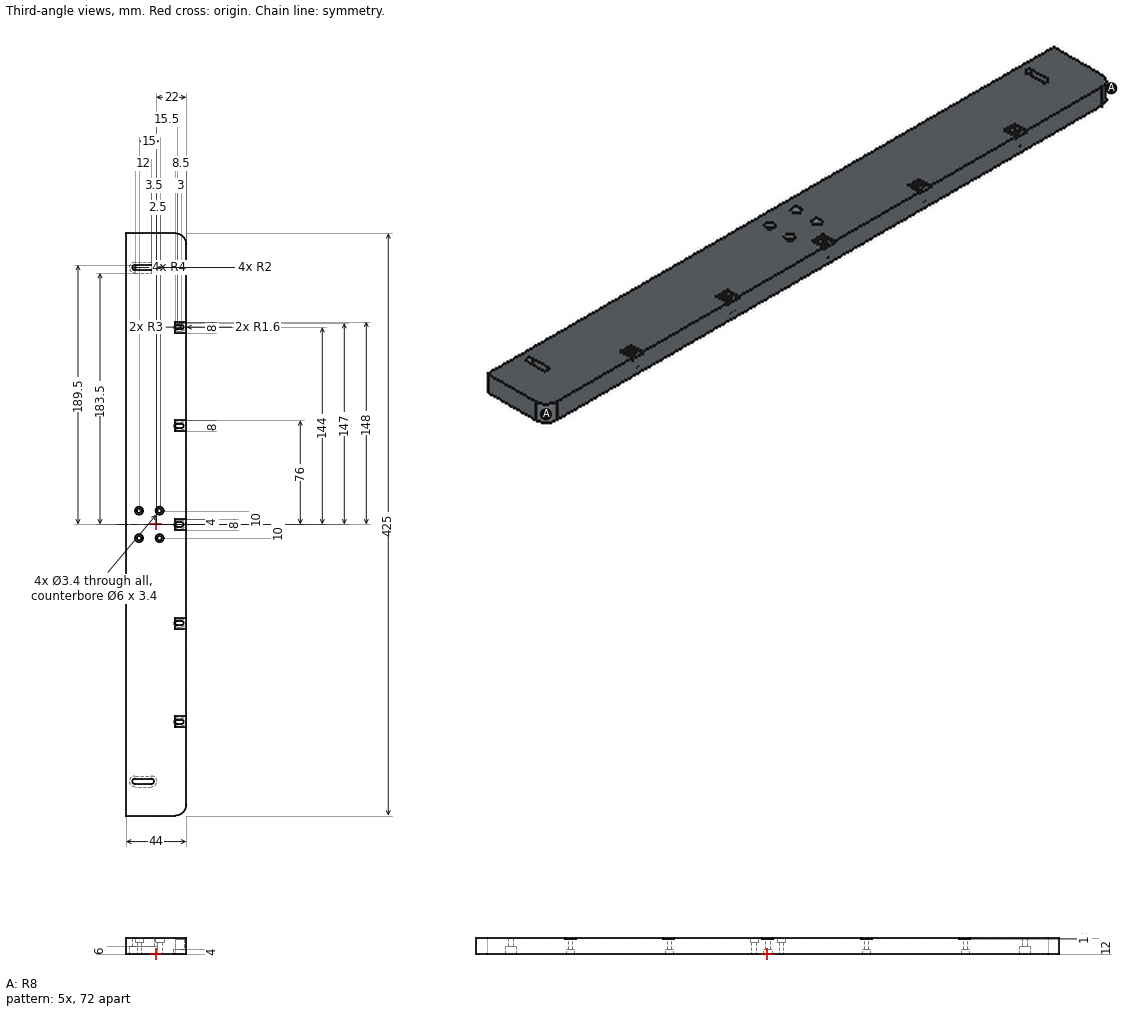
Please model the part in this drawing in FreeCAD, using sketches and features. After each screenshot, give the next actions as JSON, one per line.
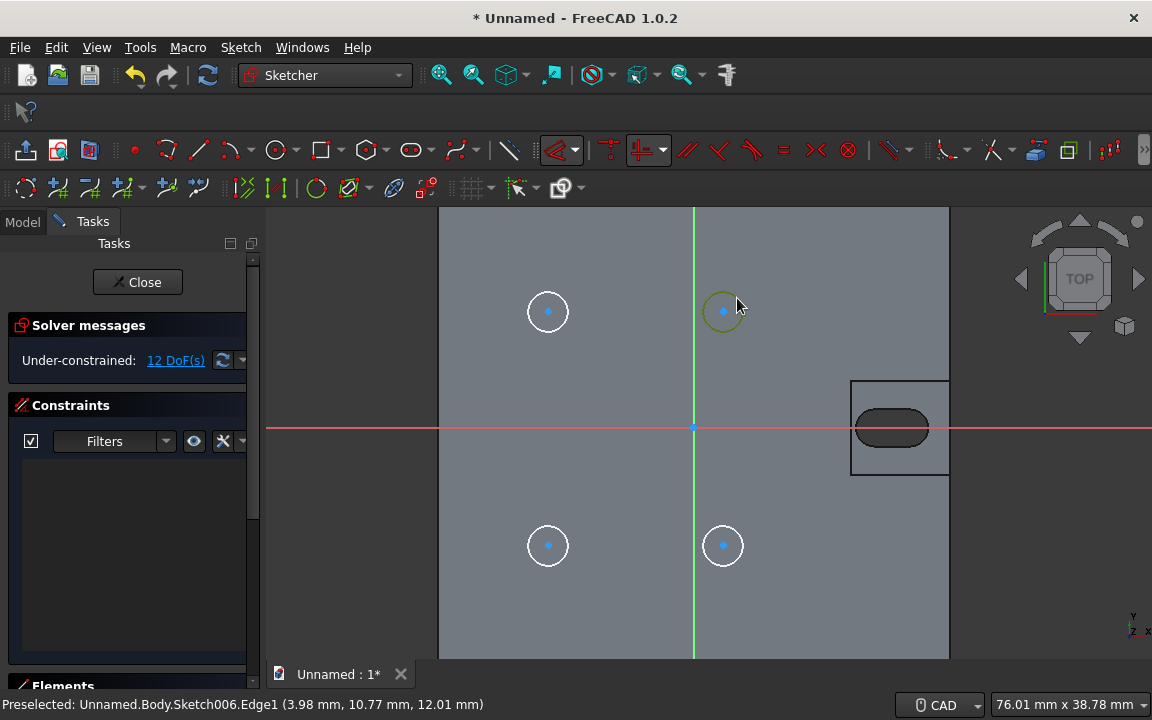
{"action": "left_click", "coordinate": [562, 298]}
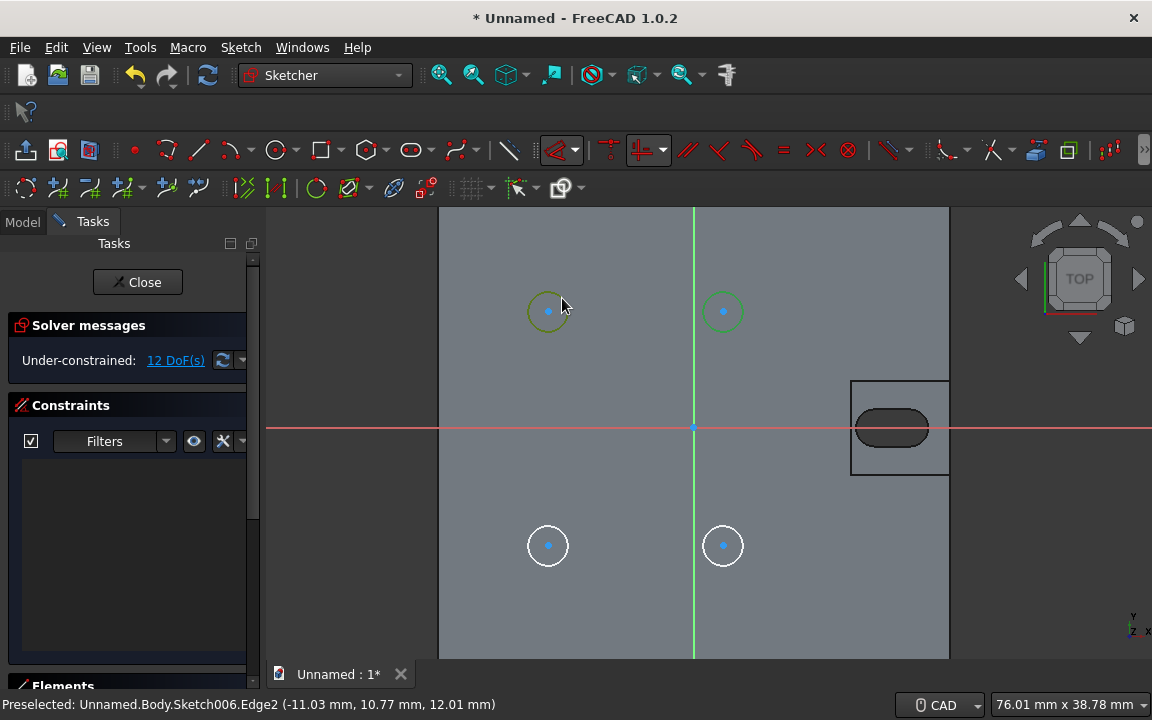
{"action": "left_click", "coordinate": [737, 532]}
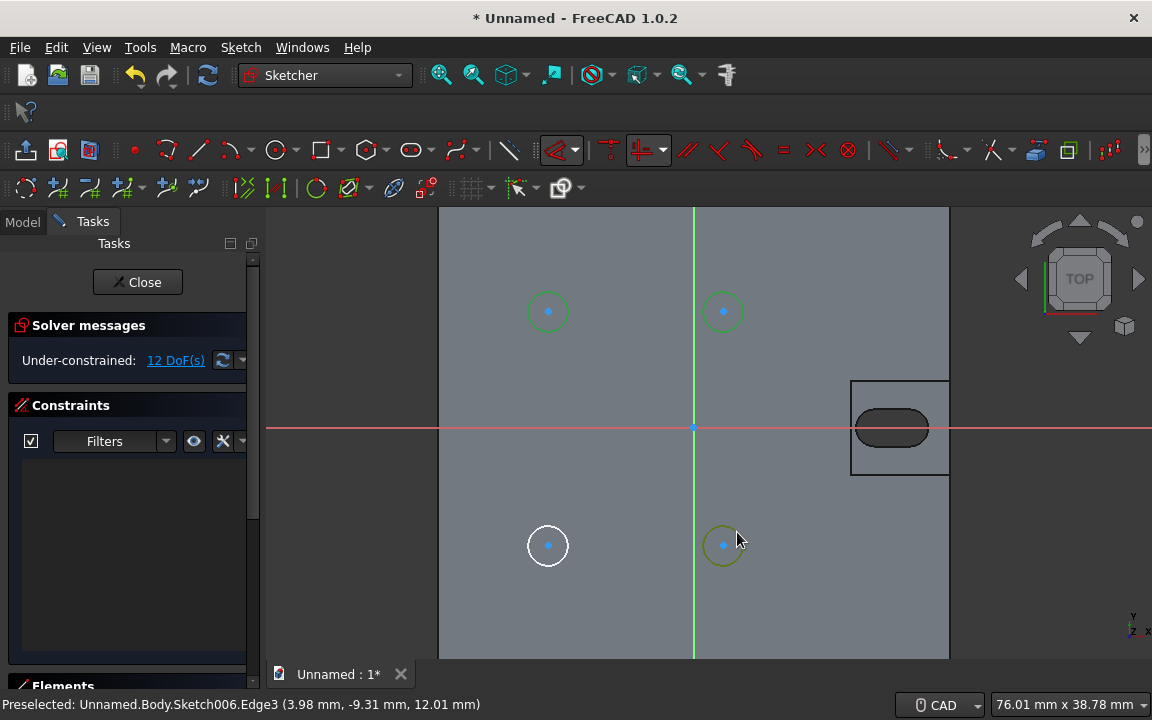
{"action": "left_click", "coordinate": [562, 532]}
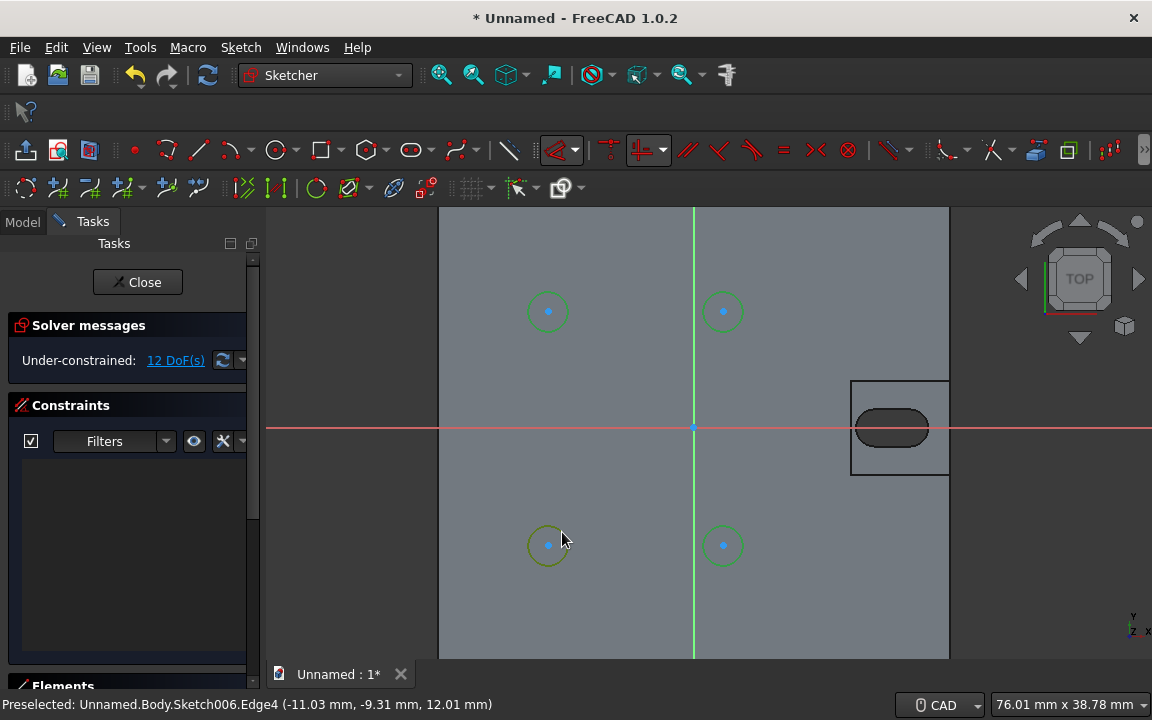
{"action": "left_click", "coordinate": [784, 150]}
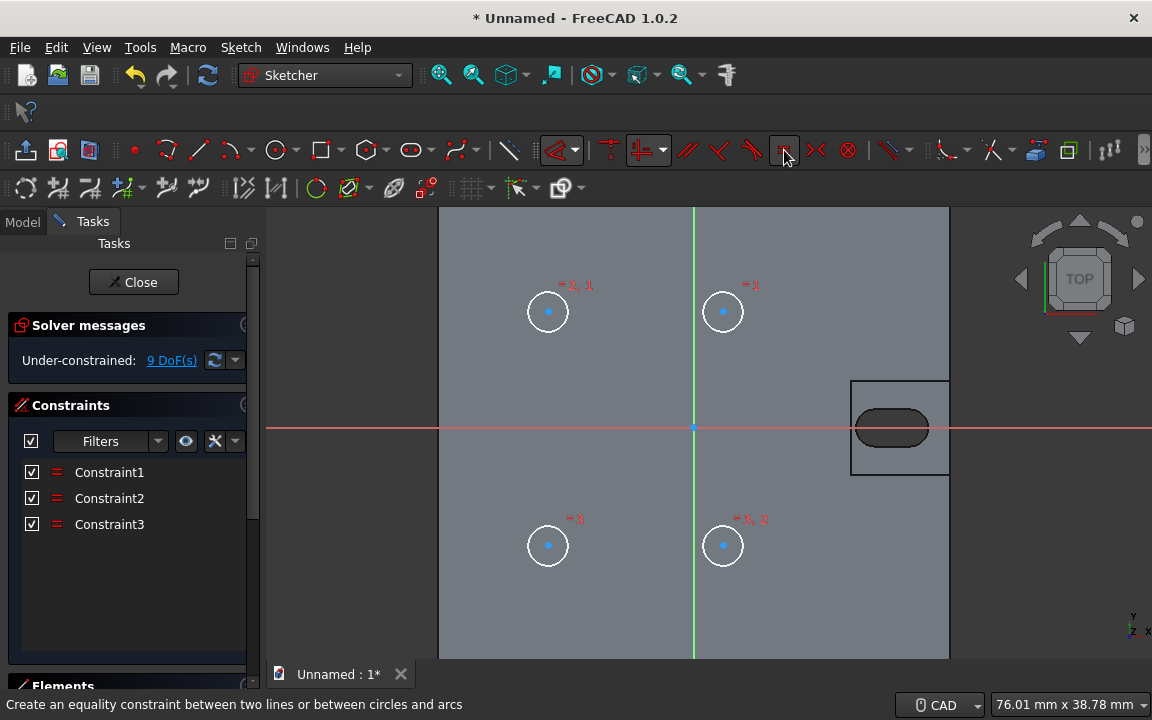
{"action": "left_click", "coordinate": [723, 312]}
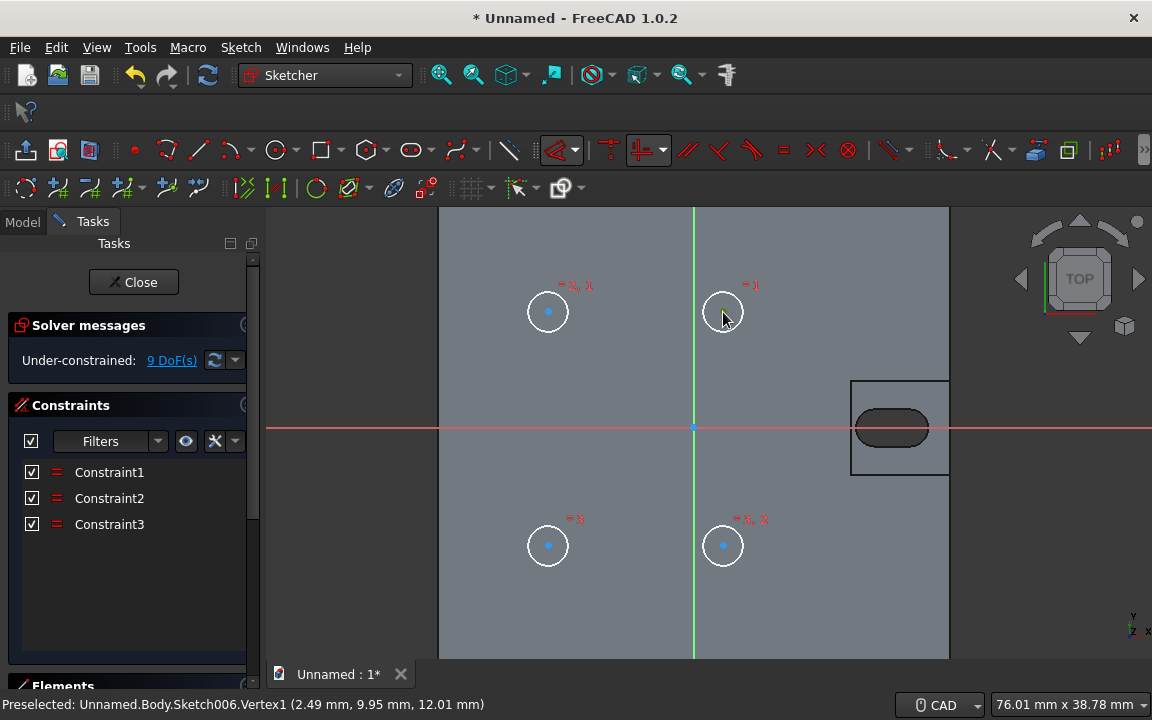
{"action": "left_click", "coordinate": [548, 312]}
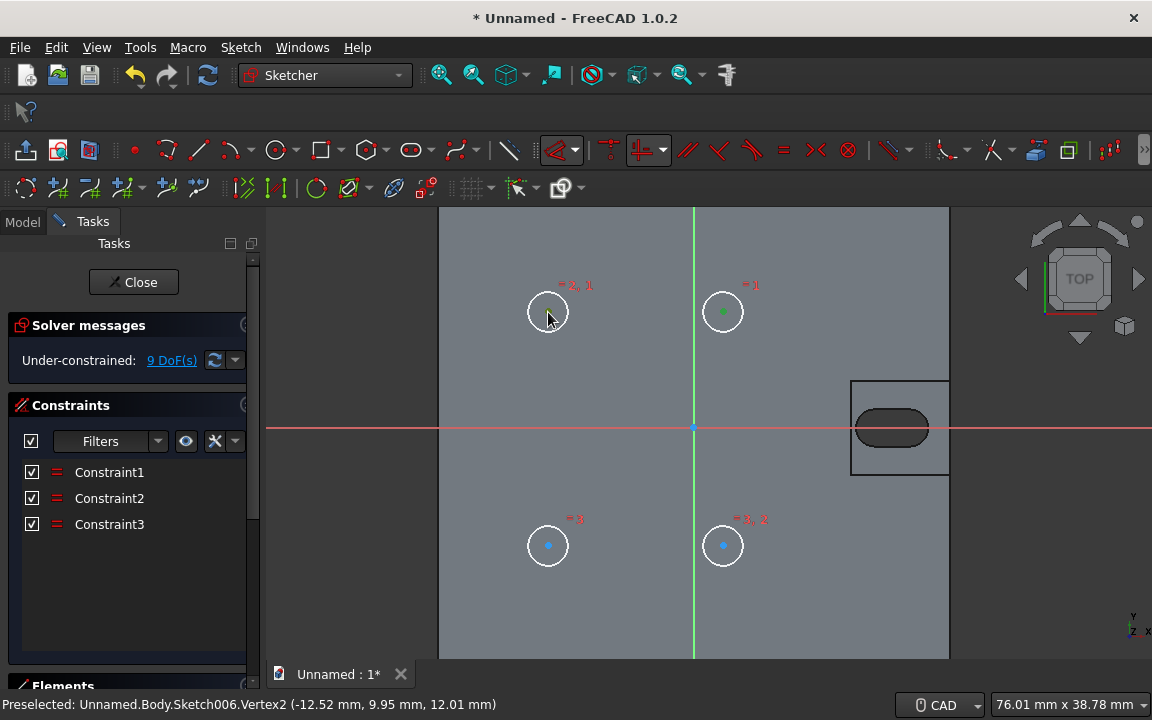
{"action": "key", "text": "h"}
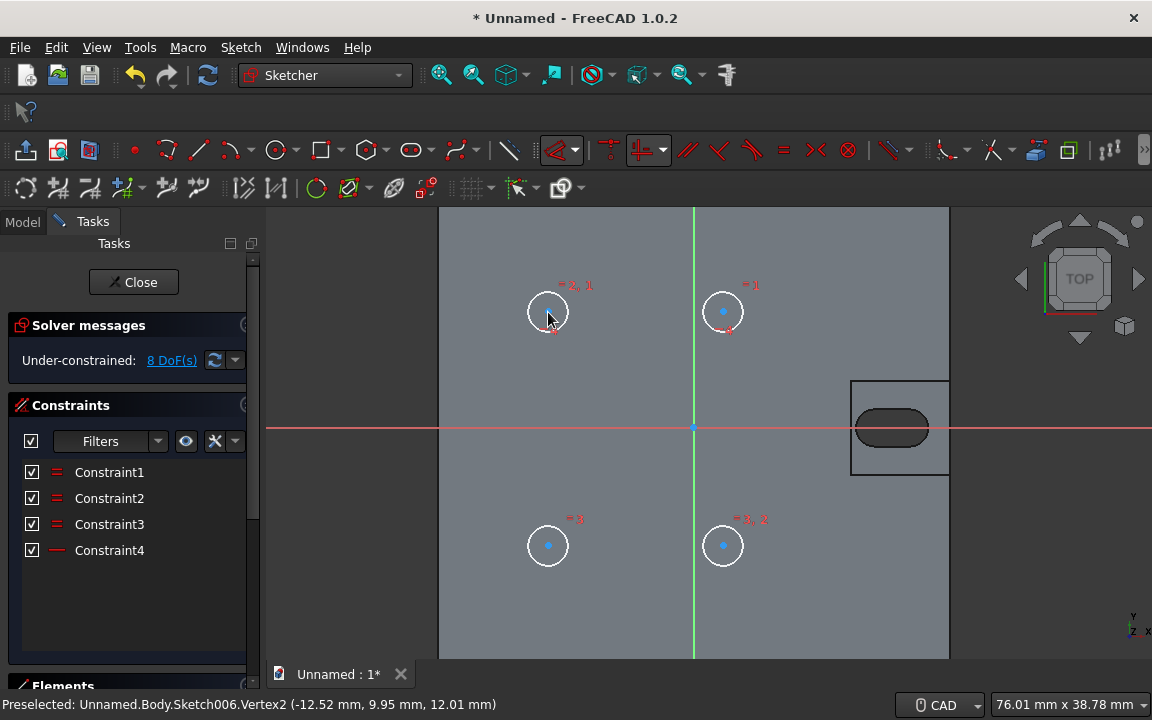
{"action": "left_click", "coordinate": [723, 312]}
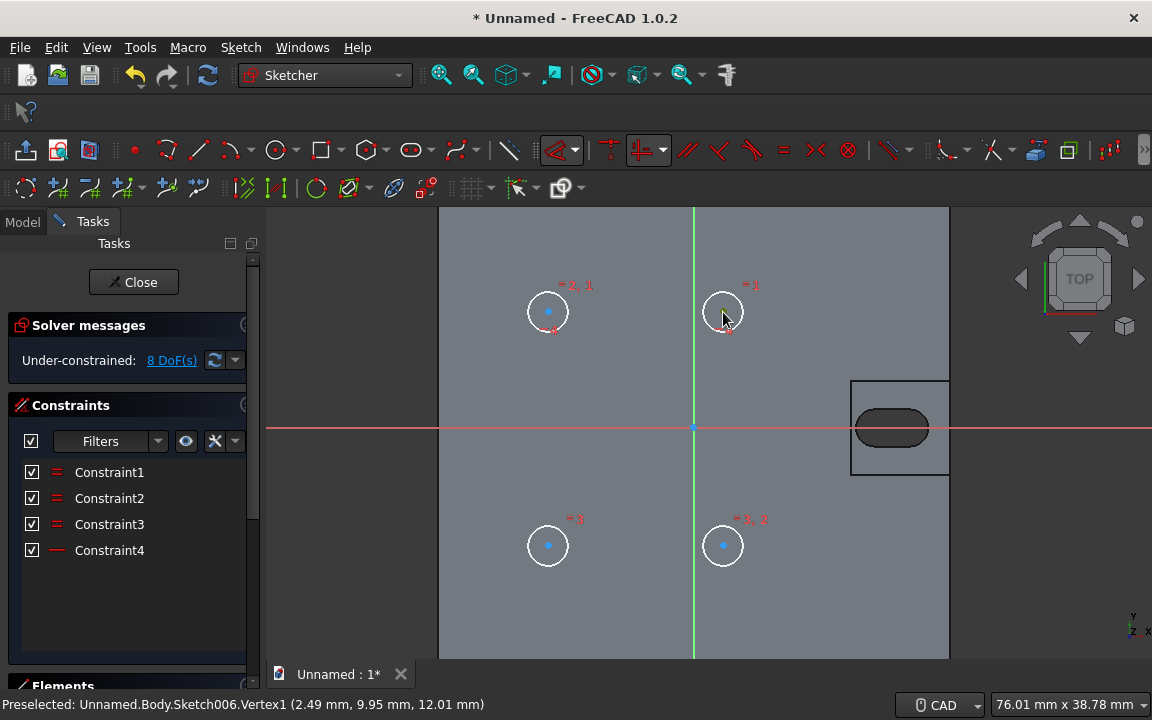
{"action": "left_click", "coordinate": [723, 546]}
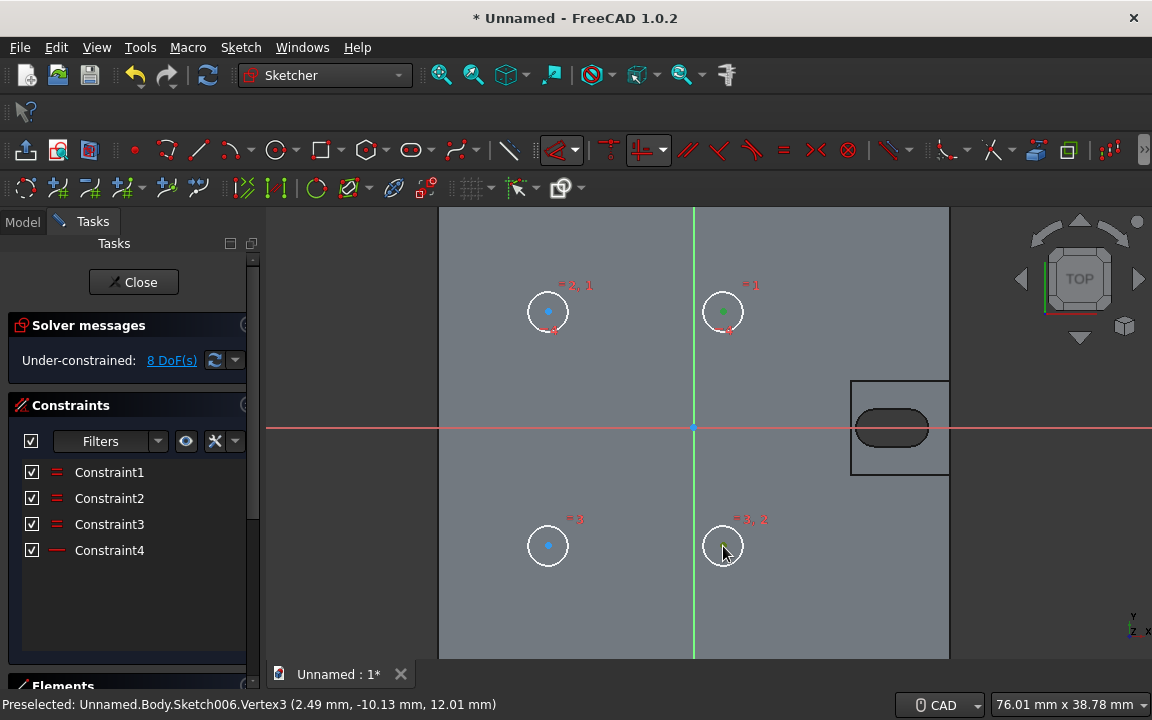
{"action": "key", "text": "v"}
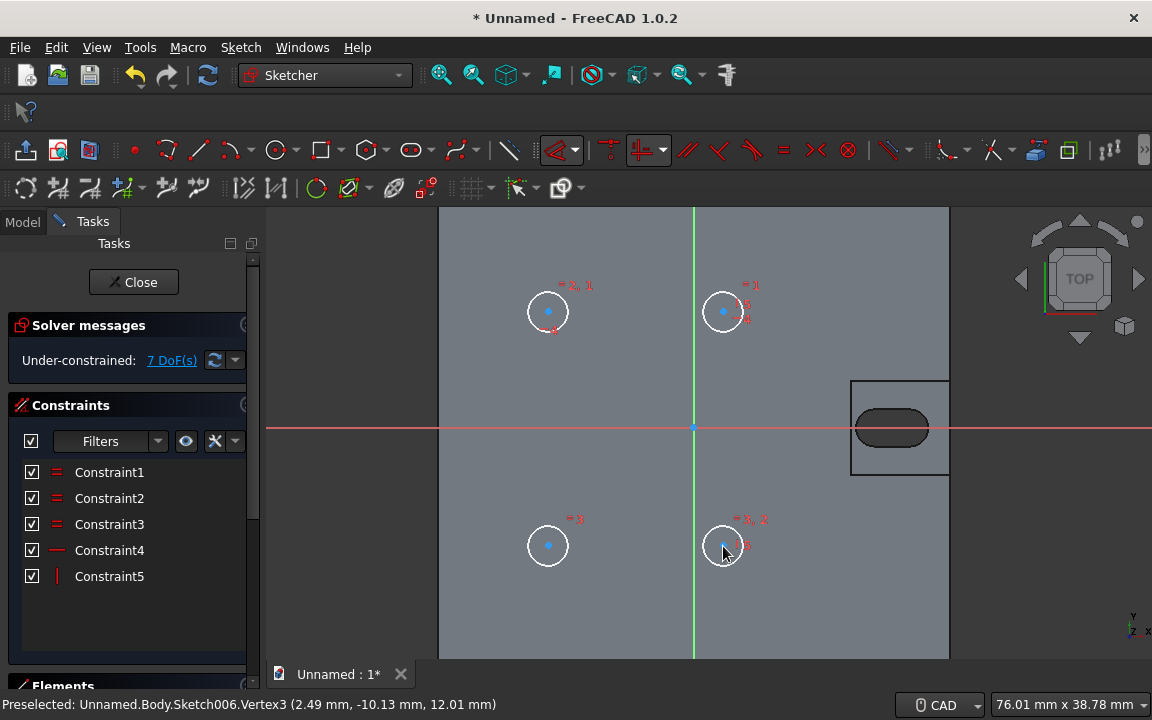
{"action": "left_click", "coordinate": [548, 312]}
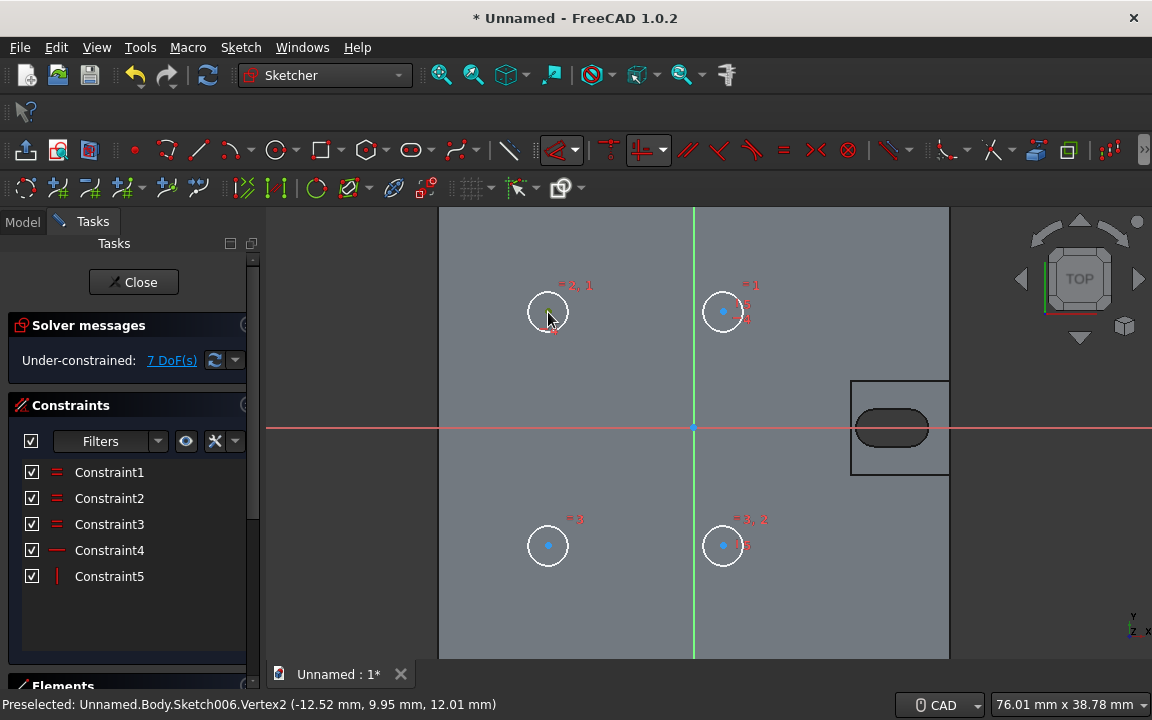
{"action": "left_click", "coordinate": [548, 546]}